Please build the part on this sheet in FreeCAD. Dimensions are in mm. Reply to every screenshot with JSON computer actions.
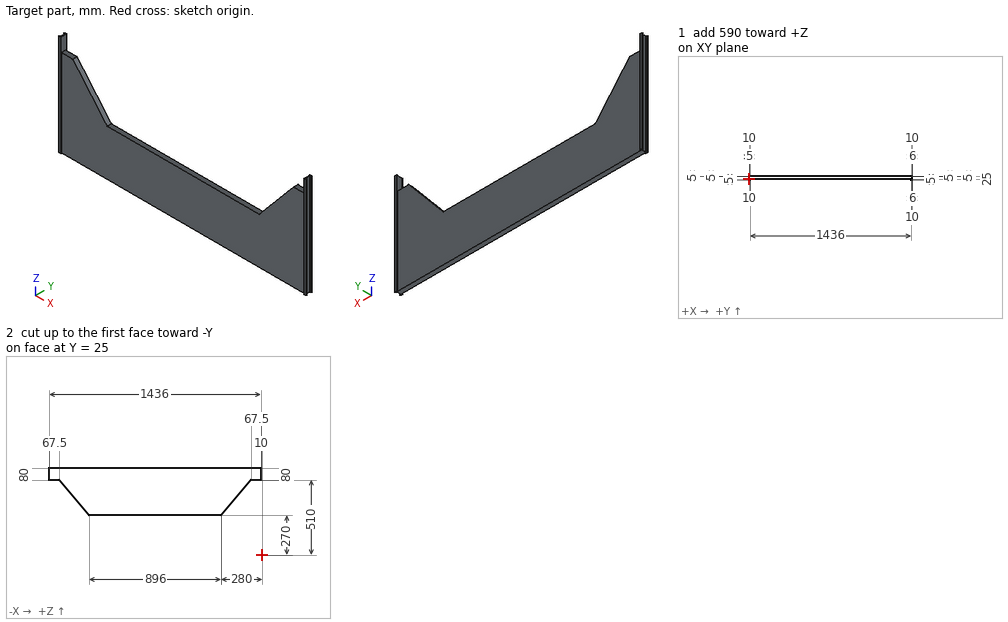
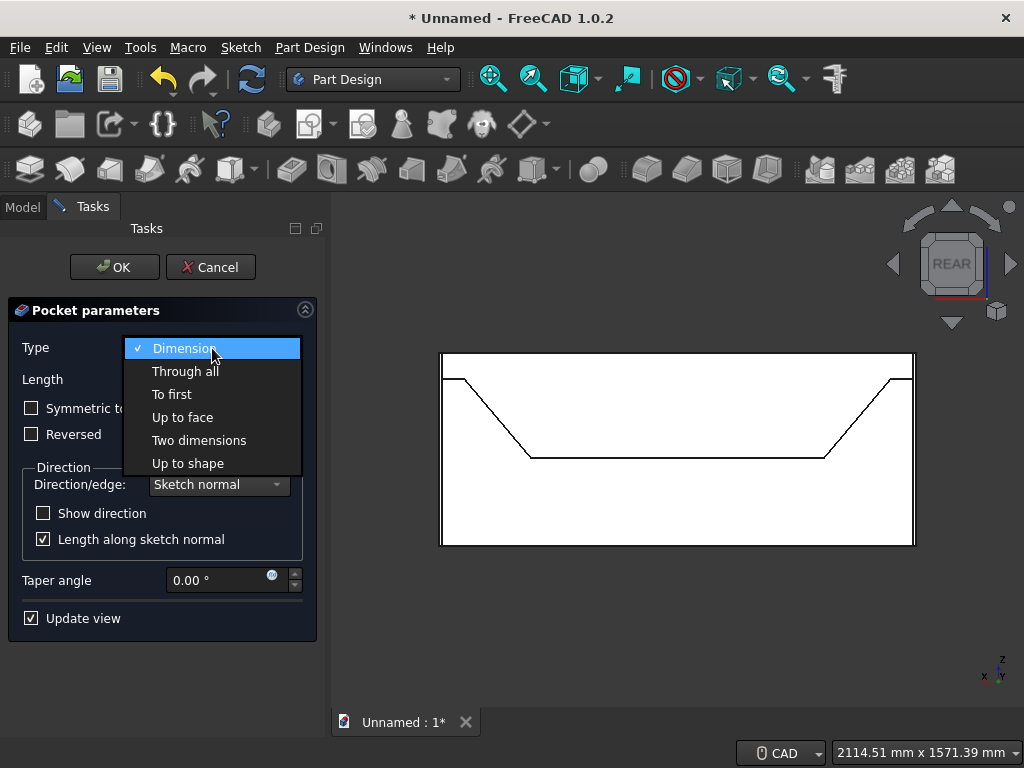
{"action": "left_click", "coordinate": [212, 394]}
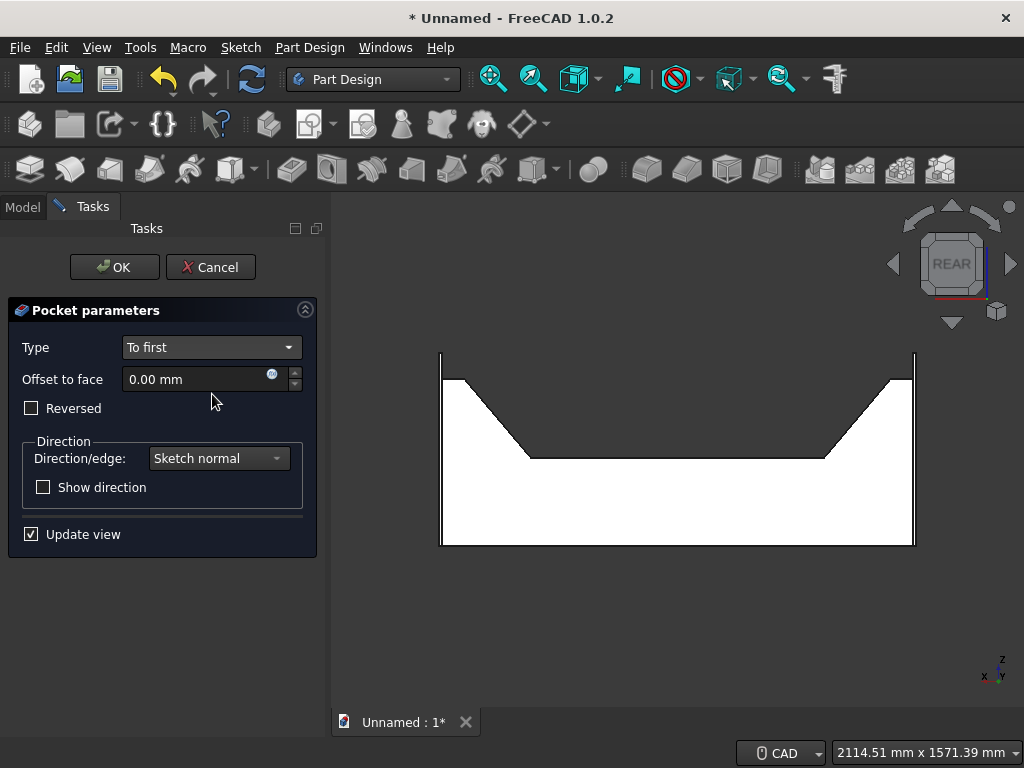
{"action": "left_click", "coordinate": [115, 267]}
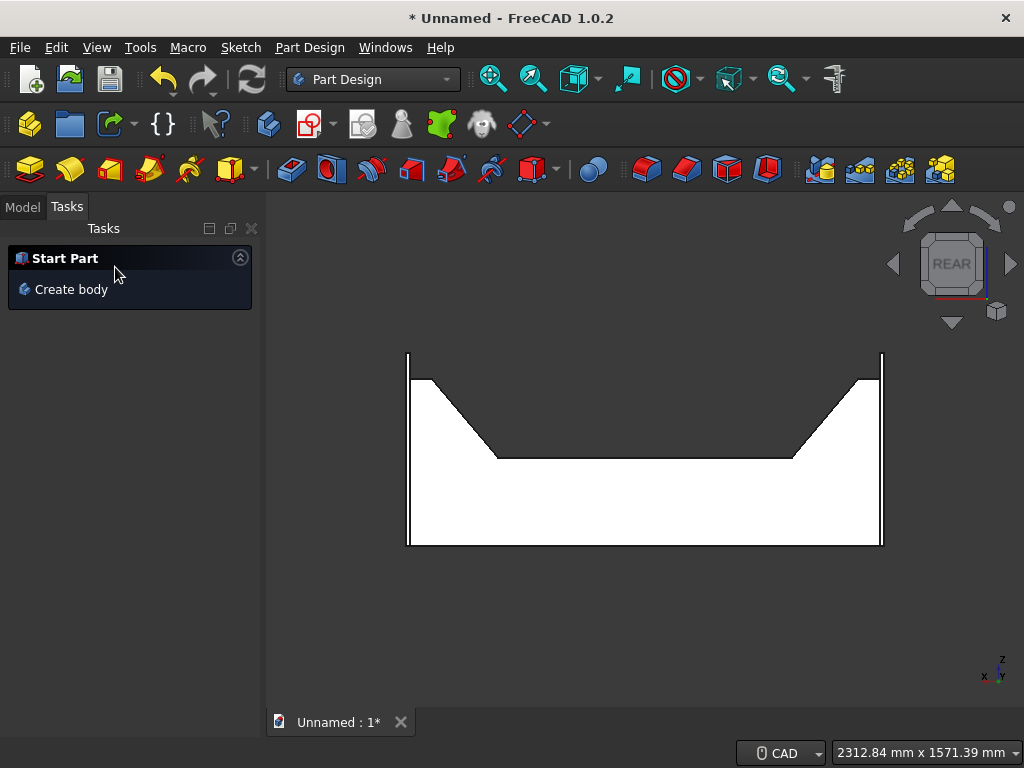
{"action": "key", "text": "0"}